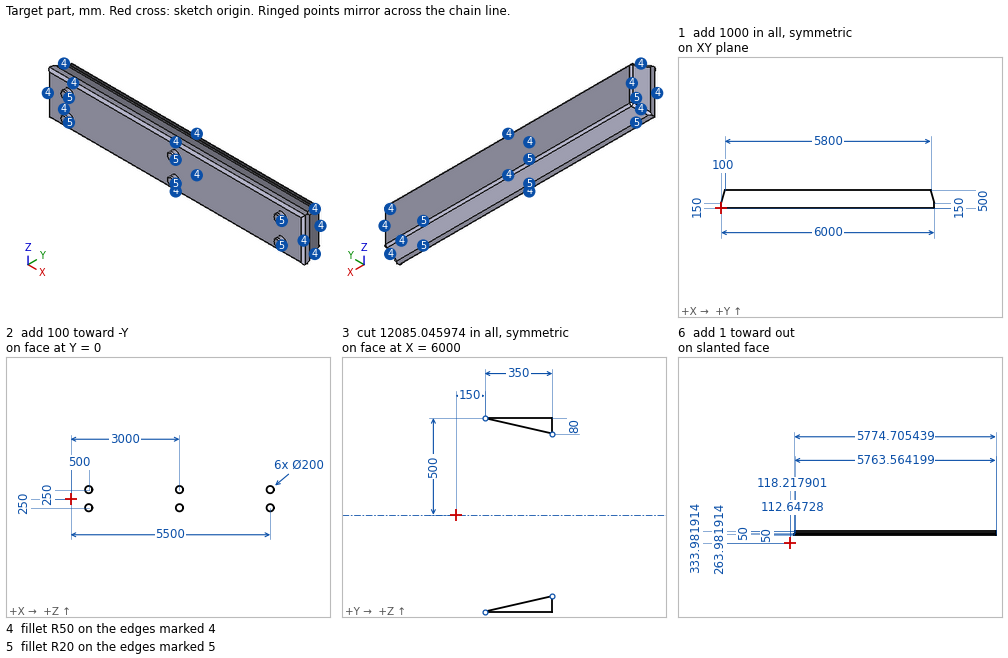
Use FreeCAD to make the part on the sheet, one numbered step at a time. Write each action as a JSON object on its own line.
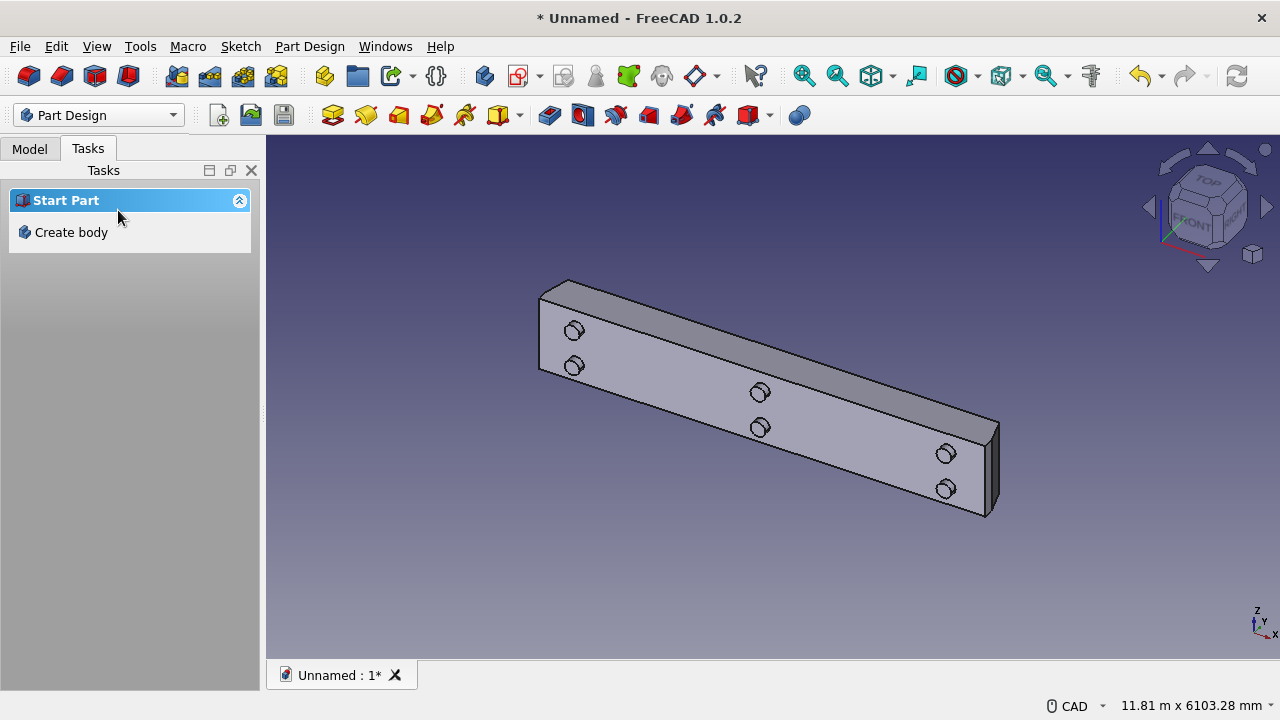
{"action": "scroll", "coordinate": [989, 457], "scroll_direction": "up", "scroll_amount": 4}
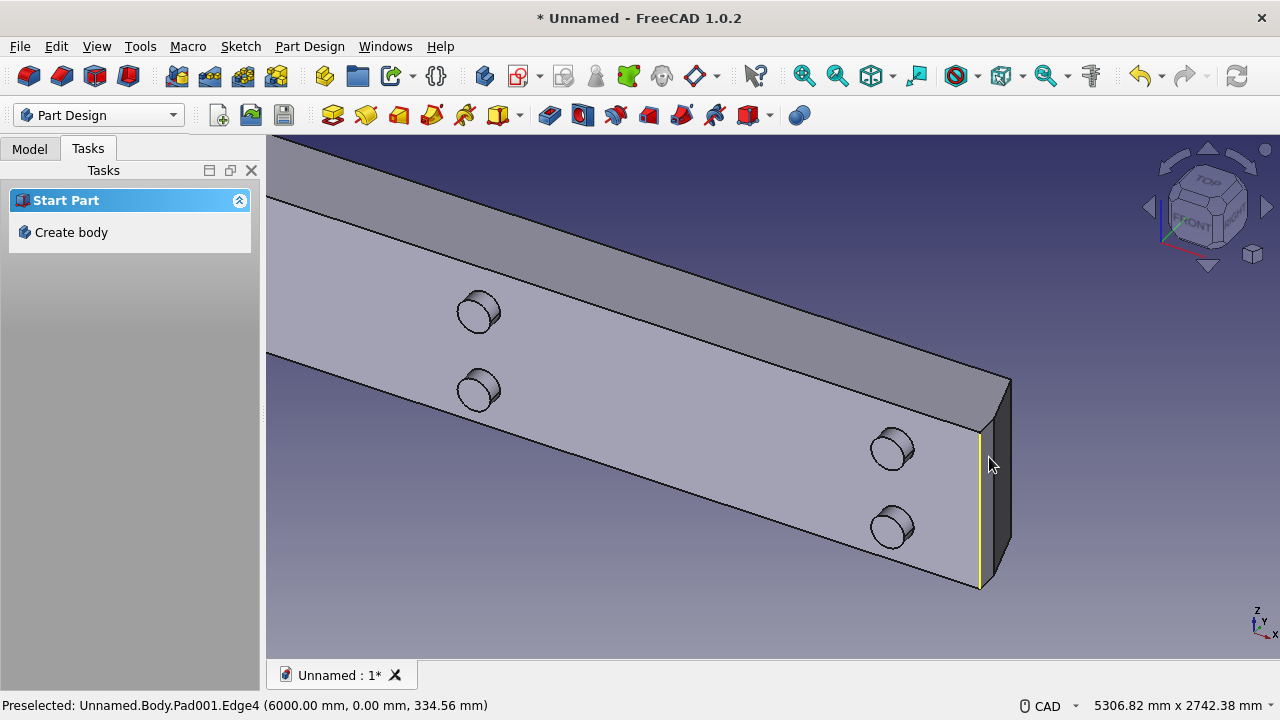
{"action": "left_click", "coordinate": [805, 76]}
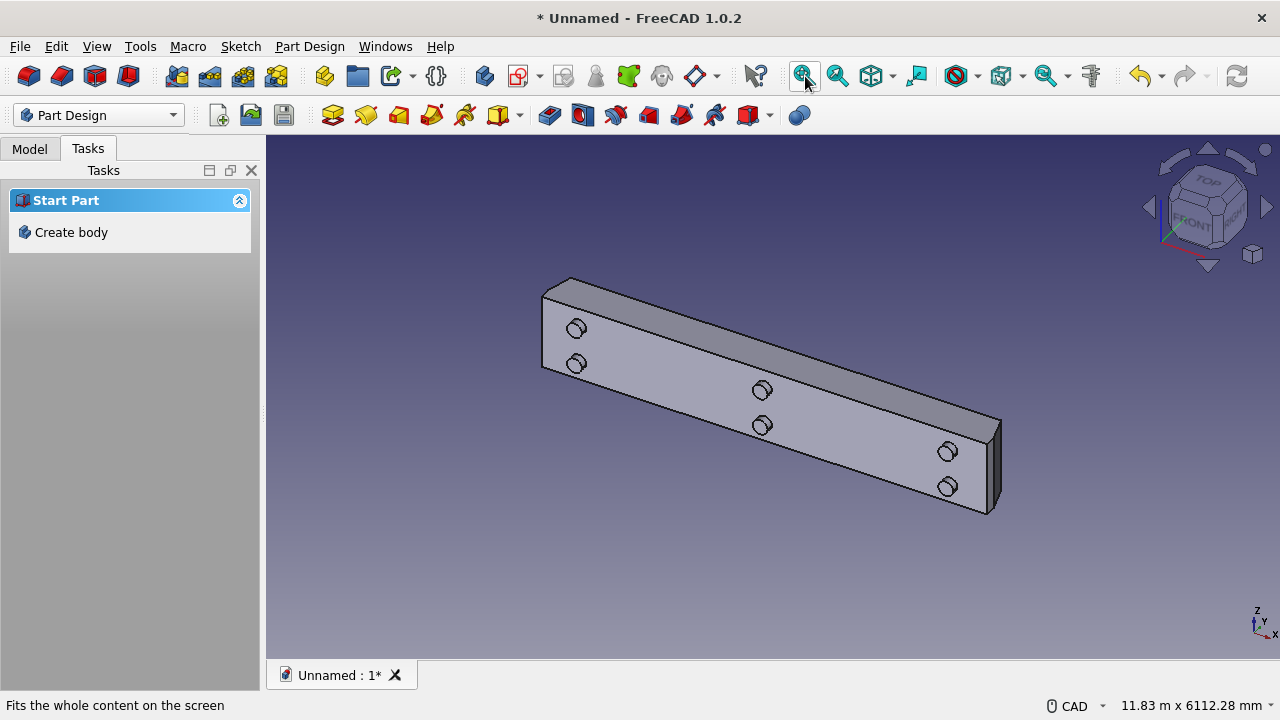
{"action": "key", "text": "0"}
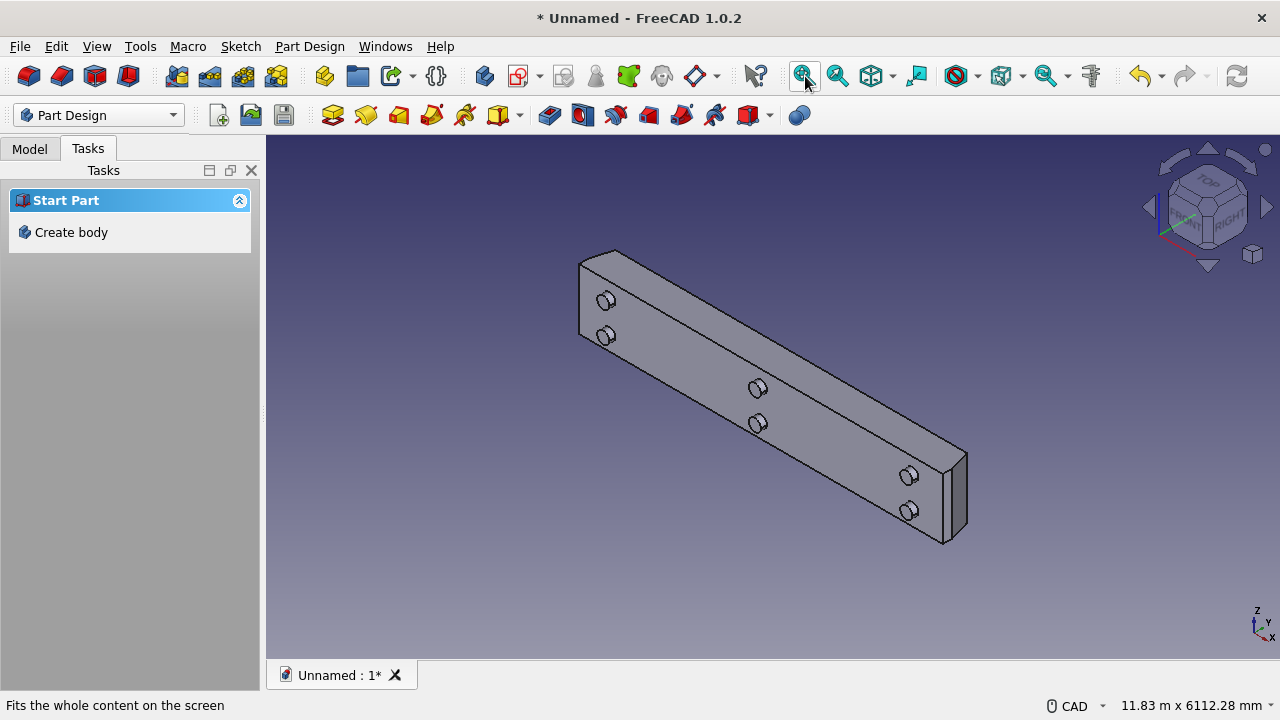
{"action": "scroll", "coordinate": [947, 485], "scroll_direction": "up", "scroll_amount": 4}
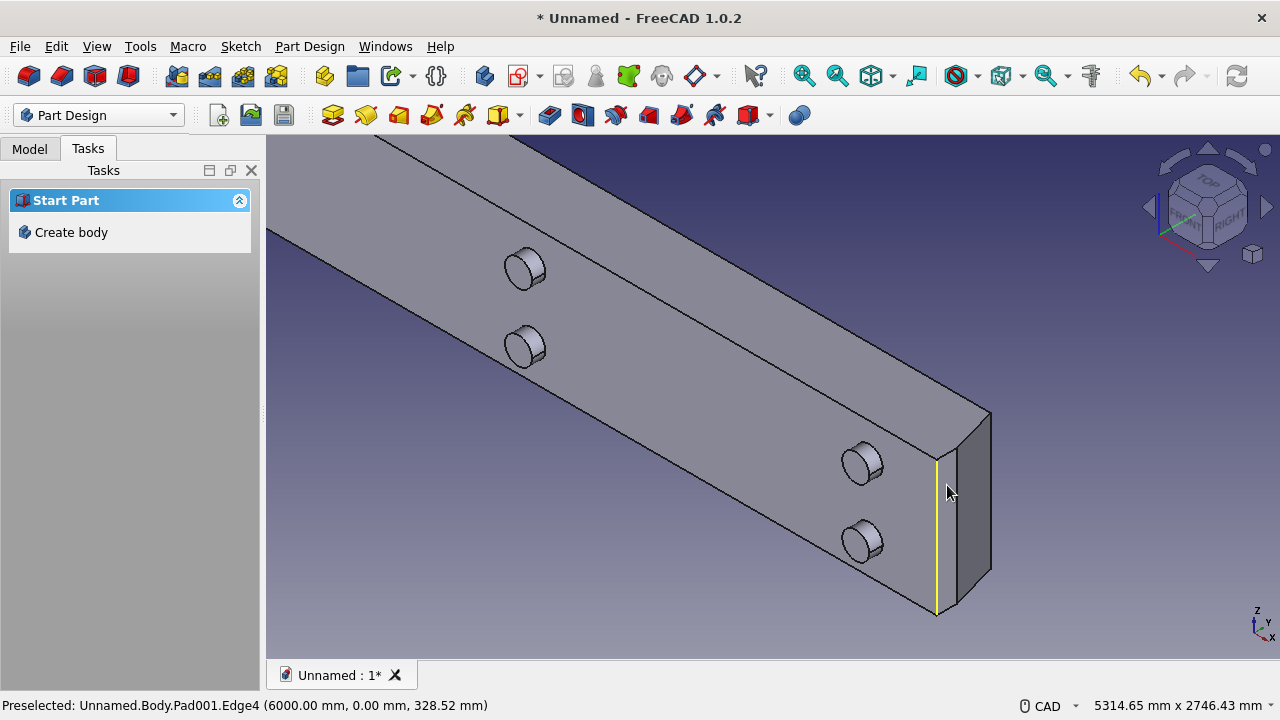
{"action": "left_click", "coordinate": [947, 486]}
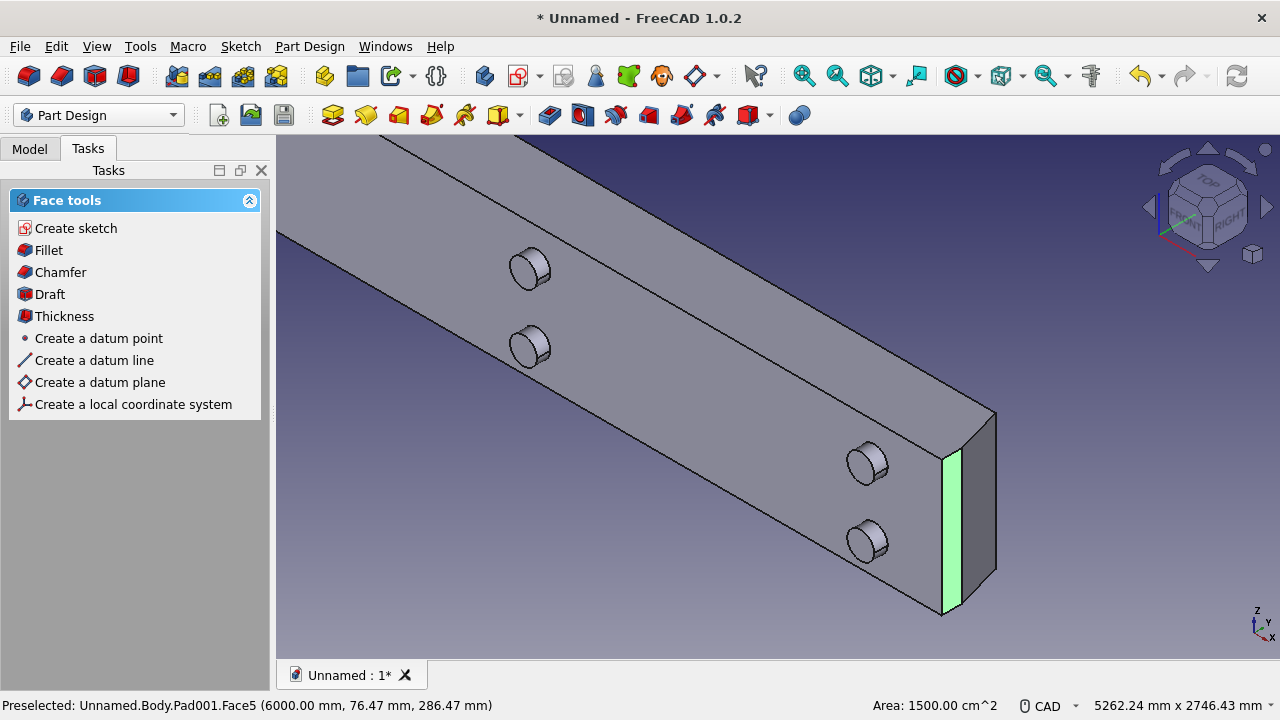
{"action": "left_click", "coordinate": [518, 76]}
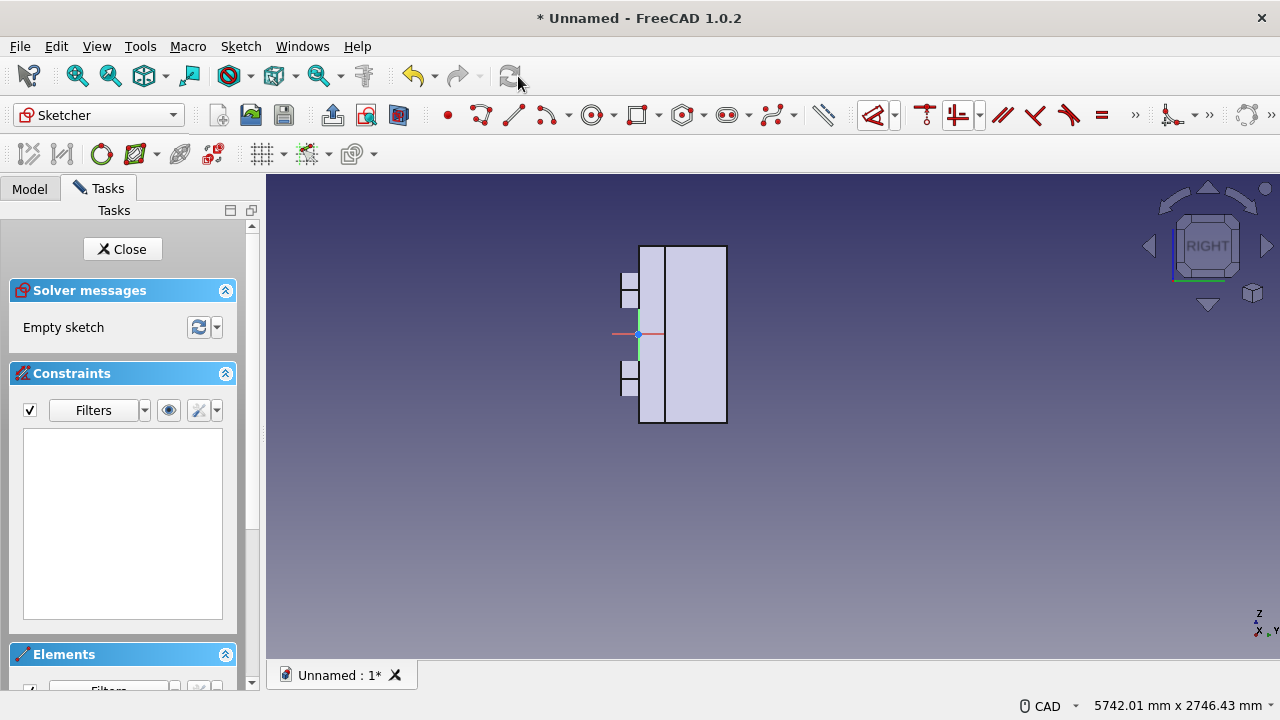
{"action": "scroll", "coordinate": [656, 234], "scroll_direction": "up", "scroll_amount": 3}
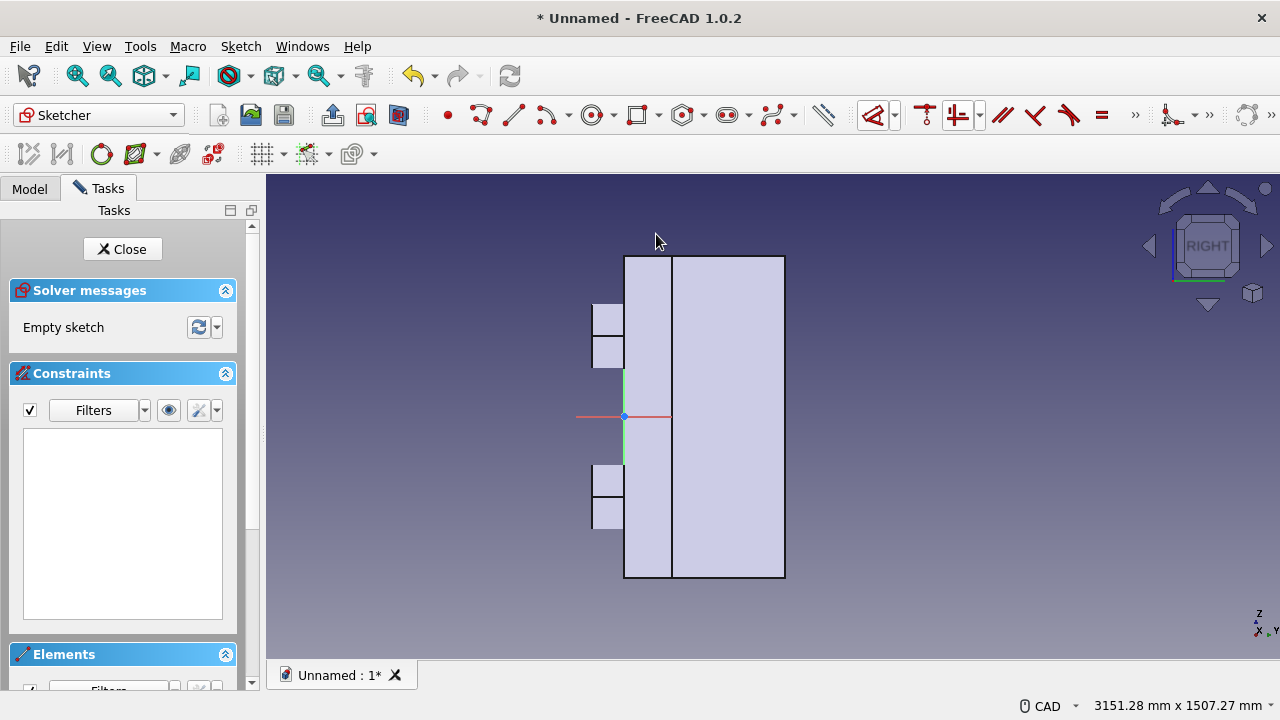
{"action": "left_click", "coordinate": [481, 116]}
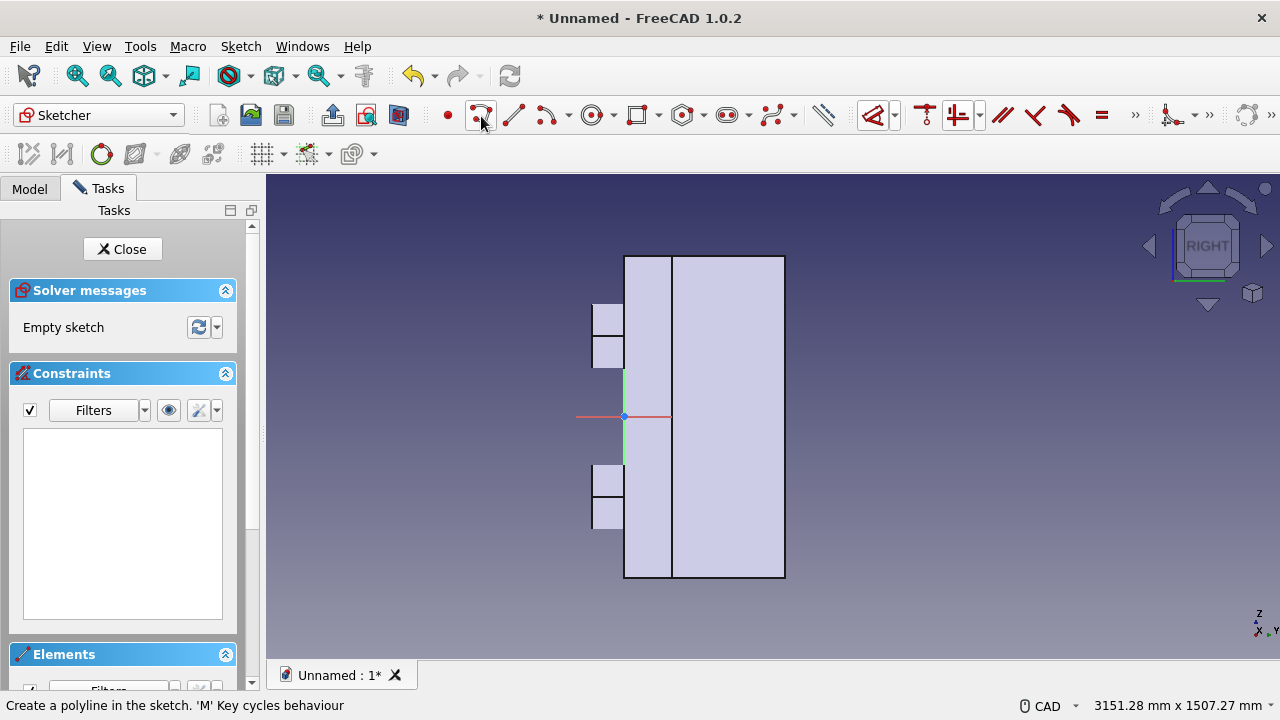
{"action": "left_click", "coordinate": [672, 256]}
{"action": "left_click", "coordinate": [785, 282]}
{"action": "left_click", "coordinate": [785, 256]}
{"action": "left_click", "coordinate": [672, 257]}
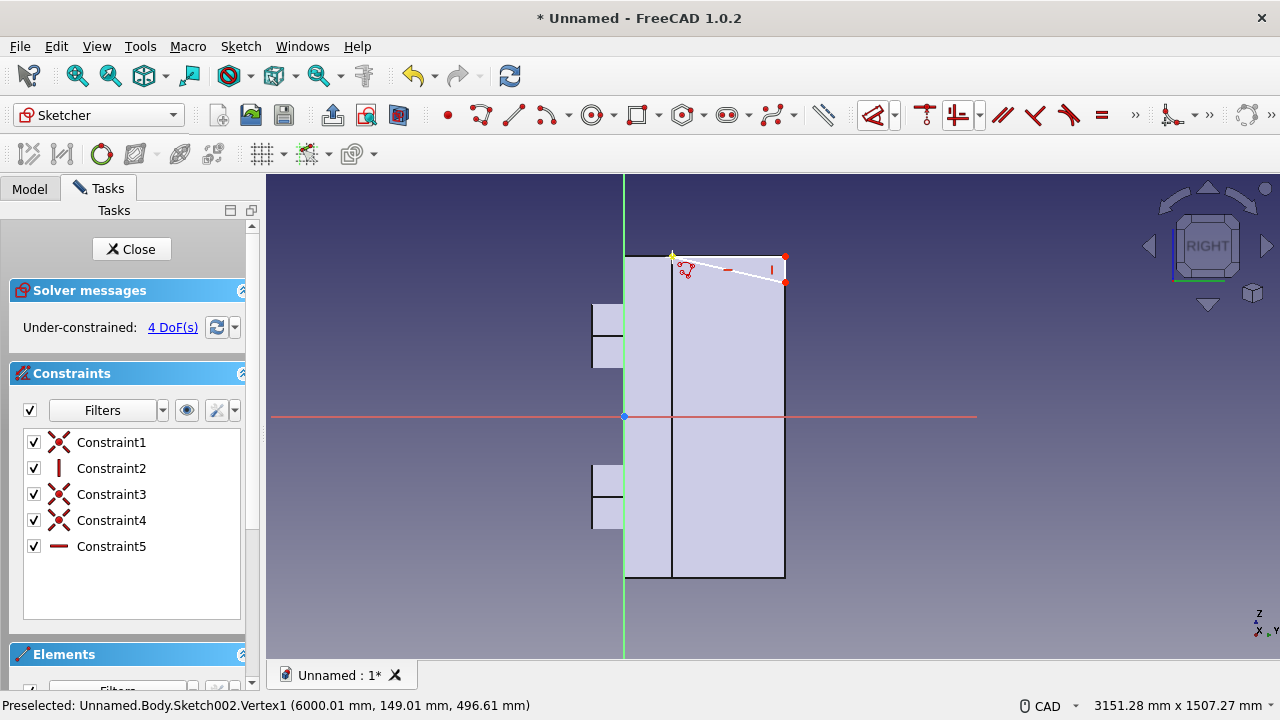
{"action": "left_click", "coordinate": [672, 578]}
{"action": "left_click", "coordinate": [785, 578]}
{"action": "left_click", "coordinate": [785, 552]}
{"action": "left_click", "coordinate": [672, 579]}
{"action": "key", "text": "Escape"}
{"action": "key", "text": "Escape"}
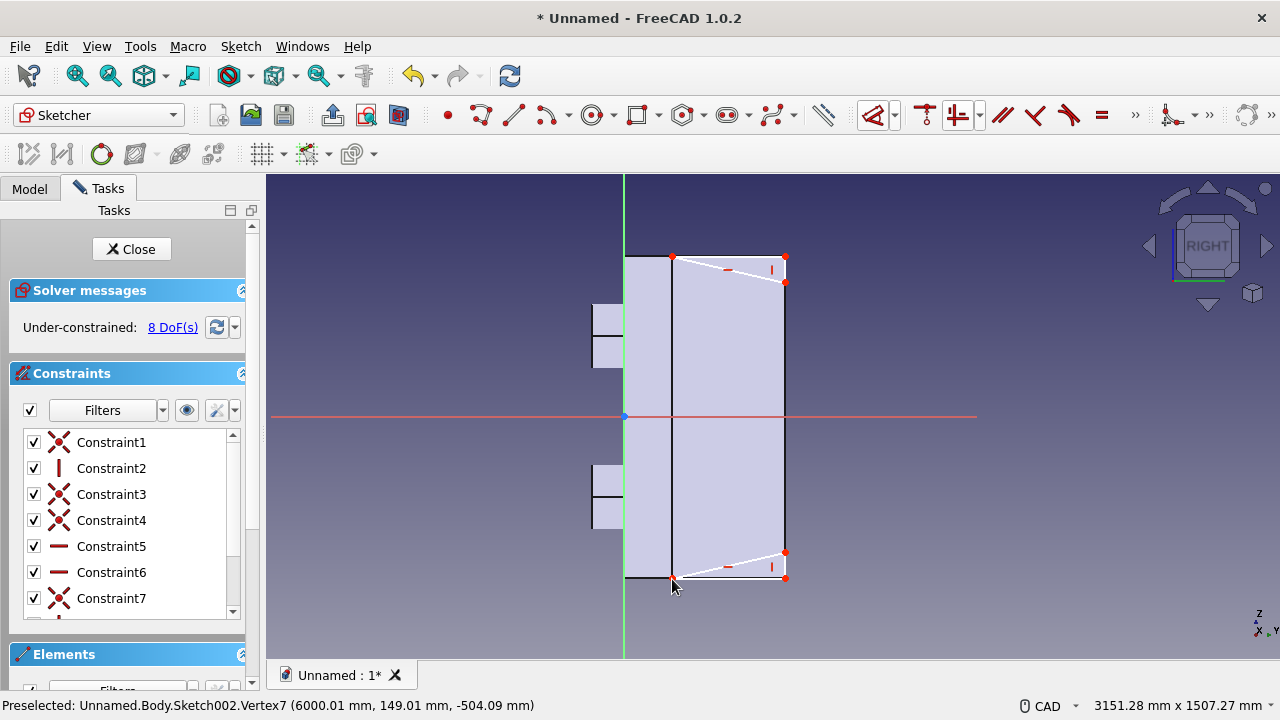
{"action": "left_click", "coordinate": [672, 257]}